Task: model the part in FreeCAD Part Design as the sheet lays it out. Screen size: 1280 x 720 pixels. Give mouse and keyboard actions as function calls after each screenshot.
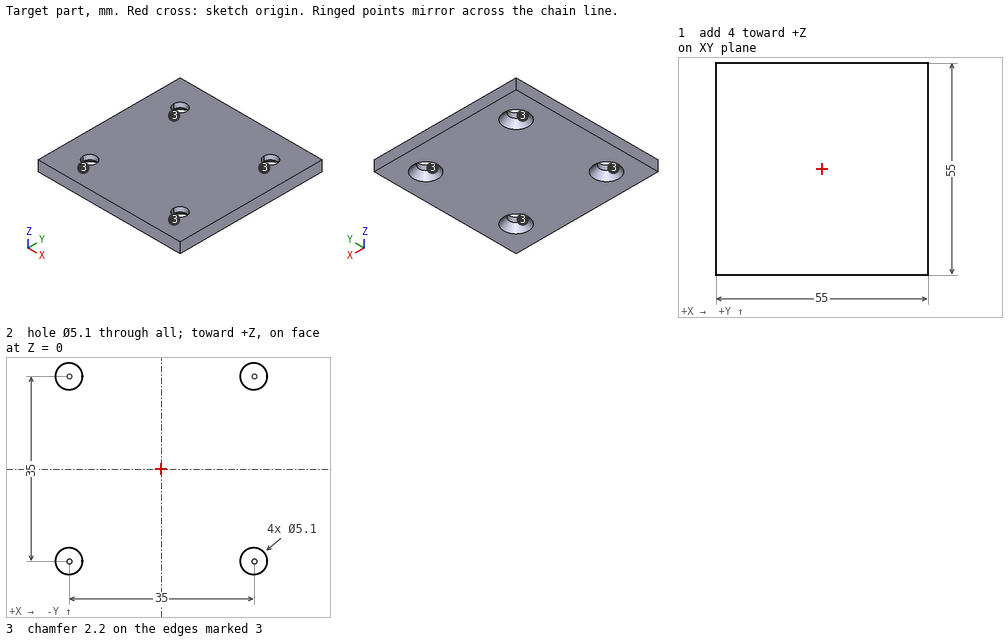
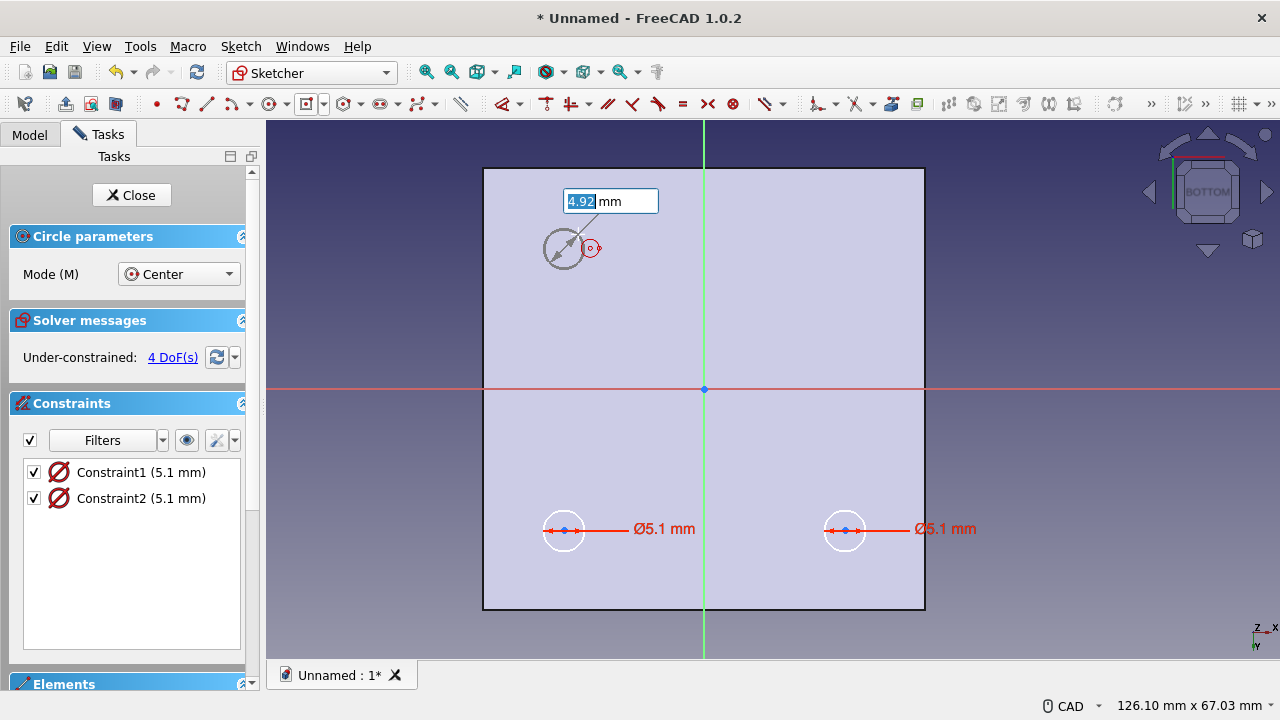
text(5.1)
key(Return)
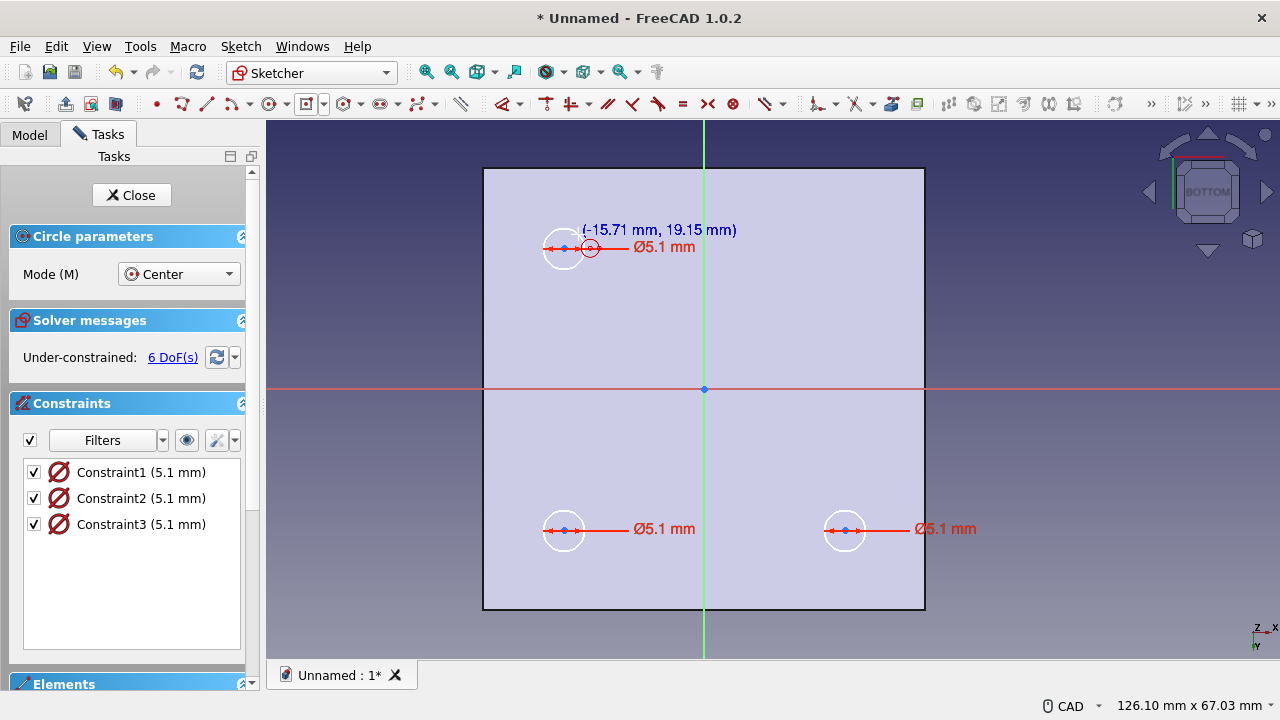
click(845, 248)
move(860, 234)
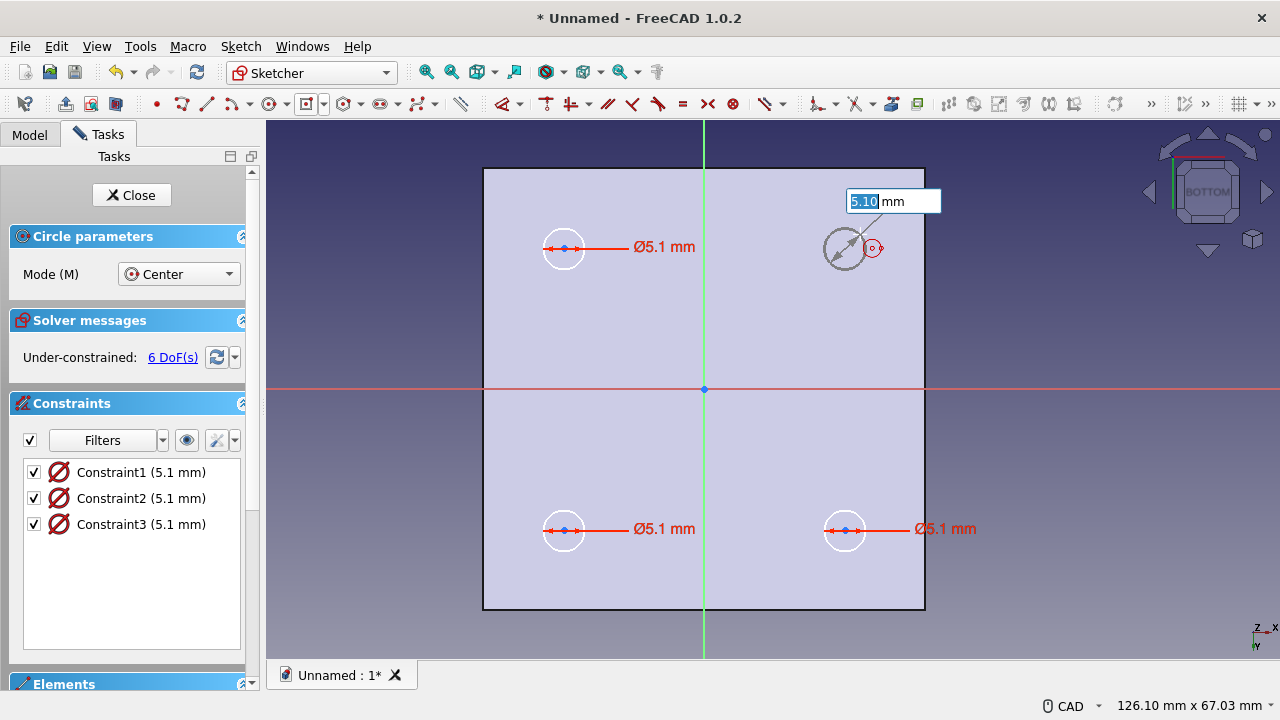
text(5.1)
key(Return)
key(Escape)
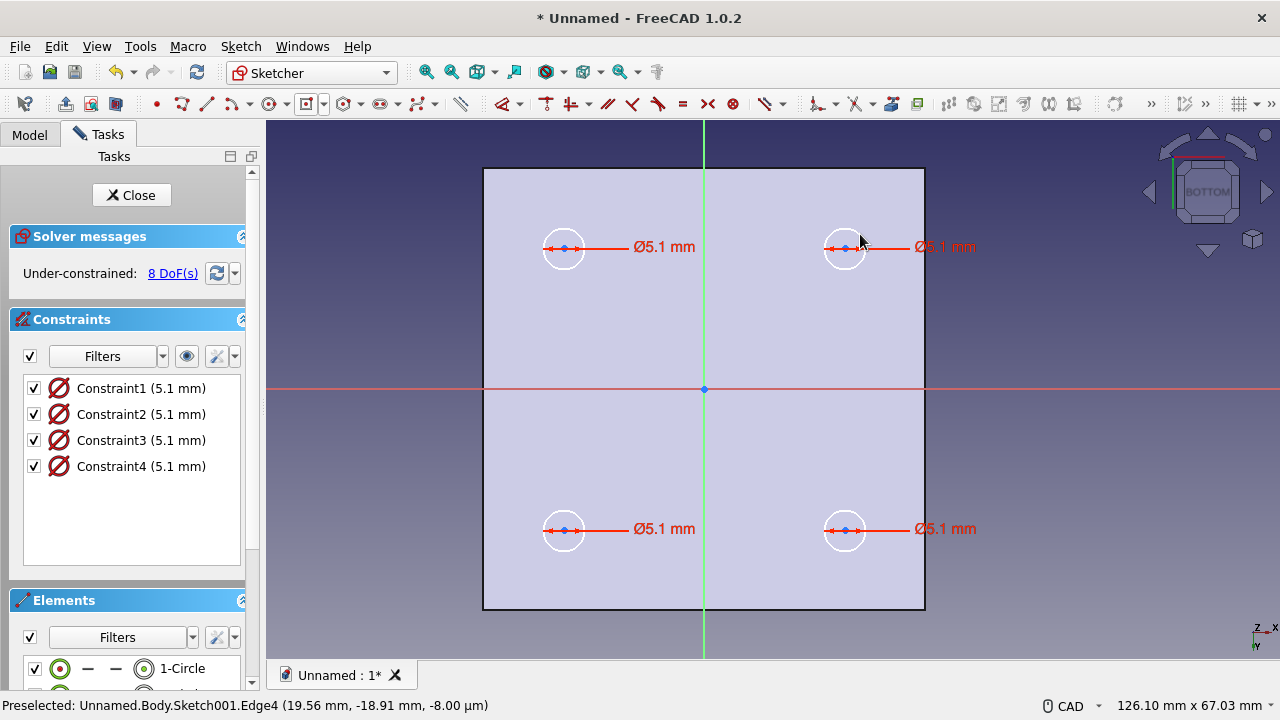
click(845, 531)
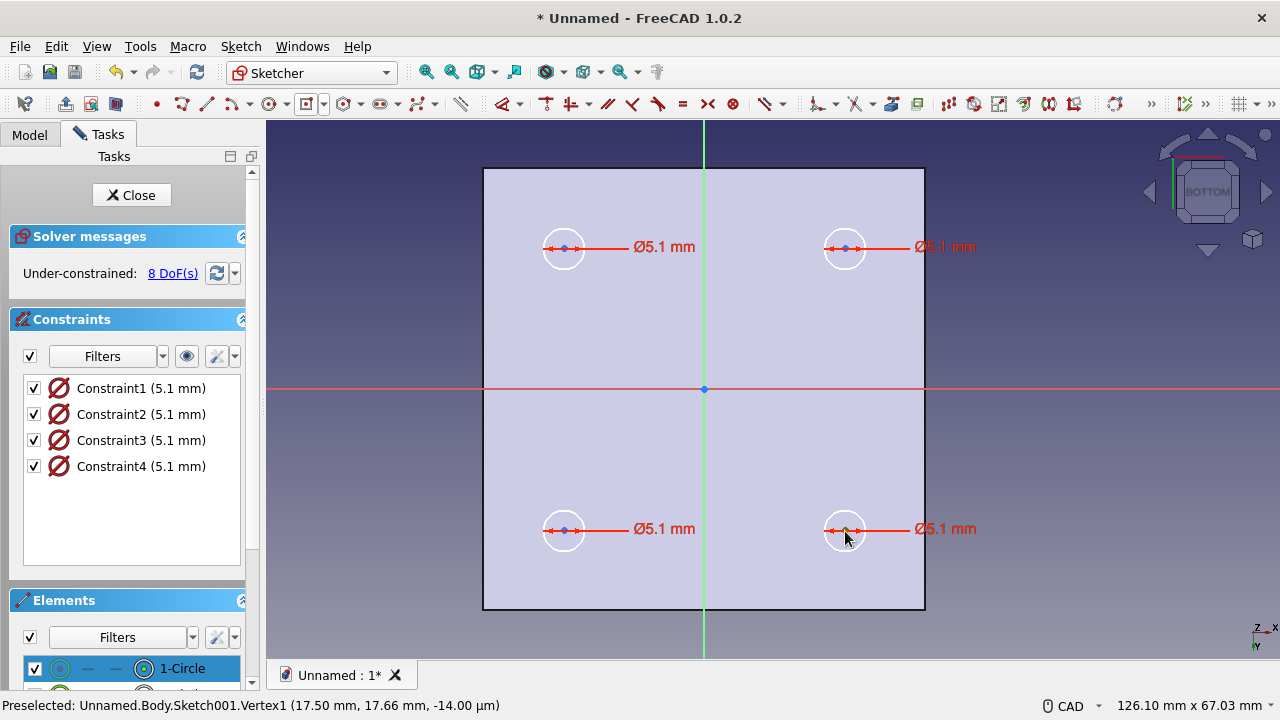
click(564, 531)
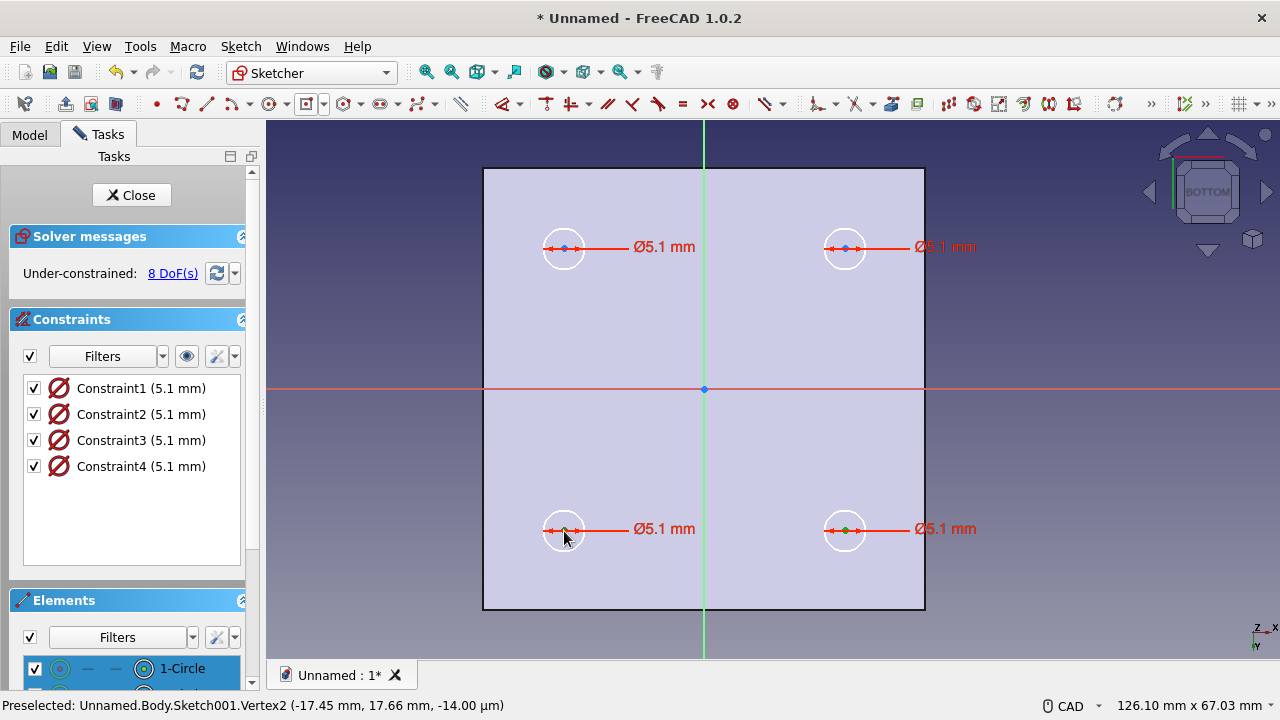
click(704, 596)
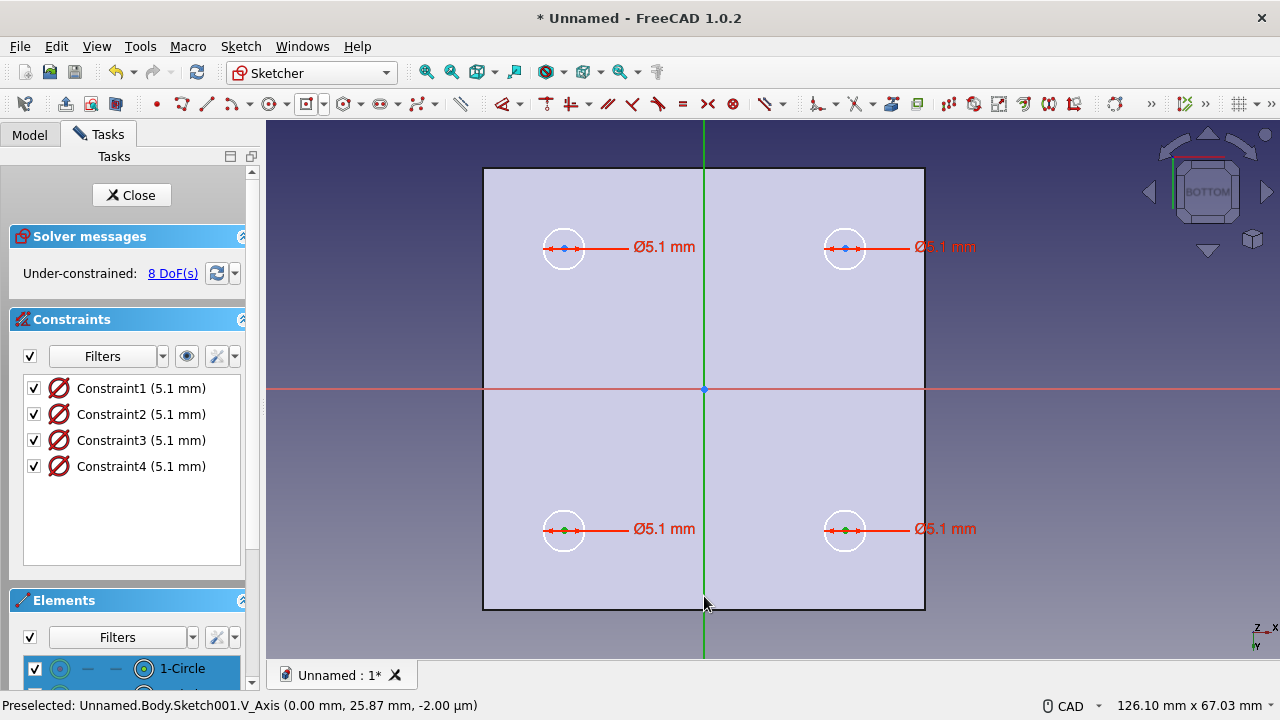
click(708, 104)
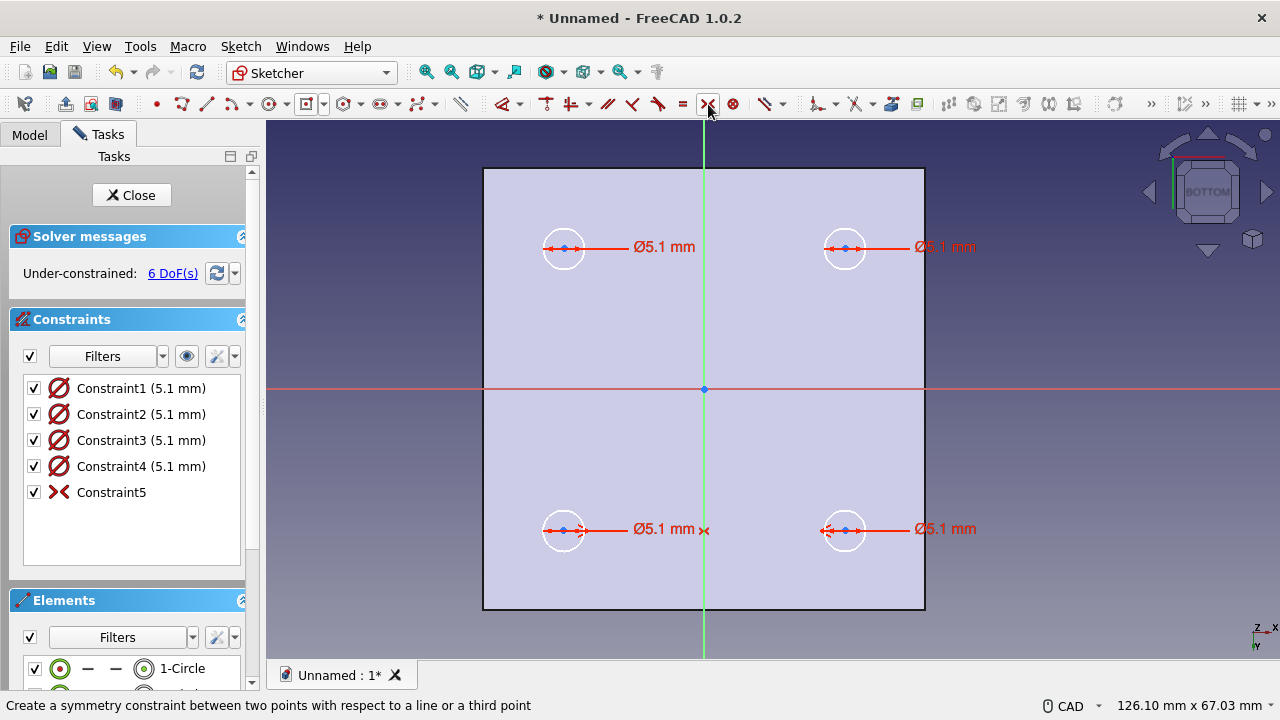
click(564, 531)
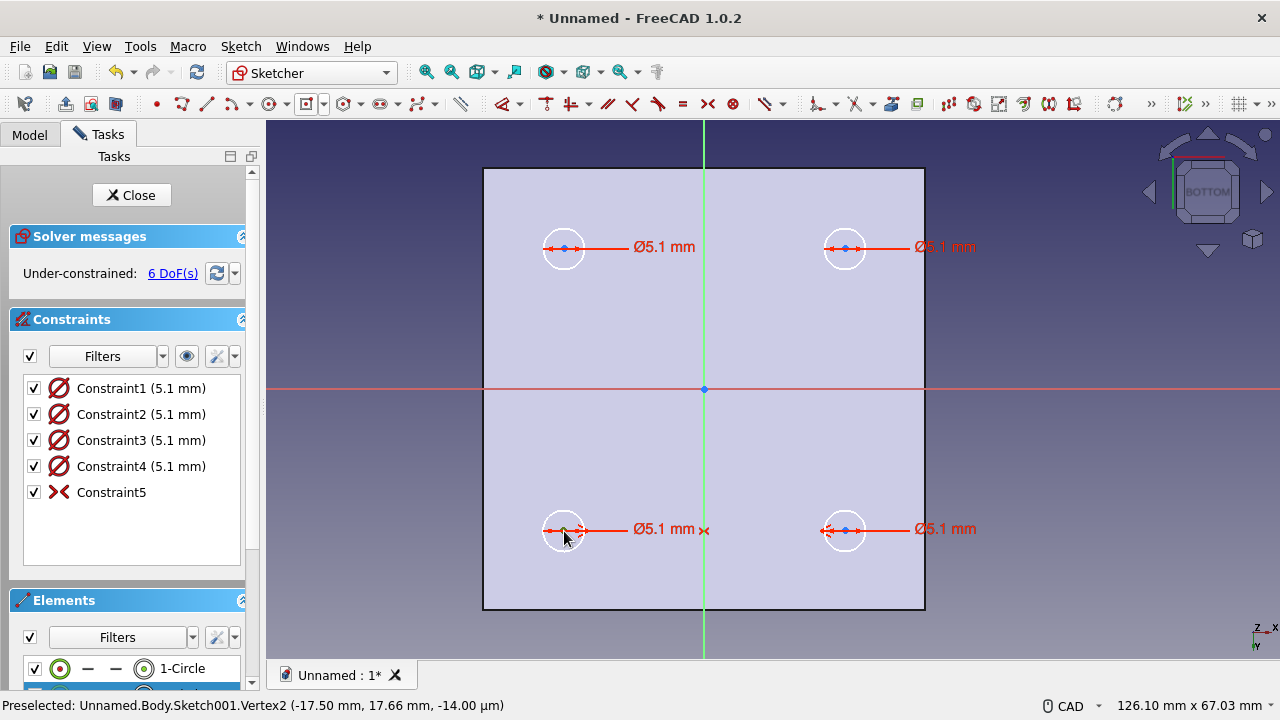
click(564, 249)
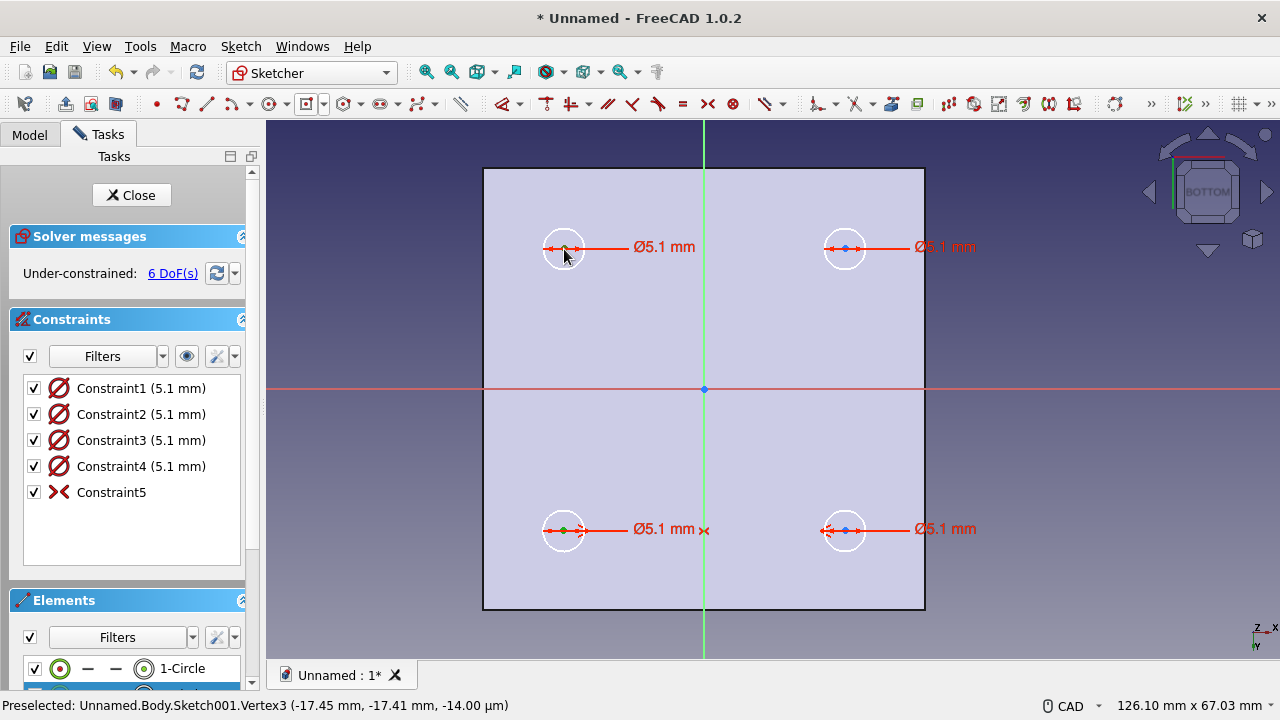
click(353, 389)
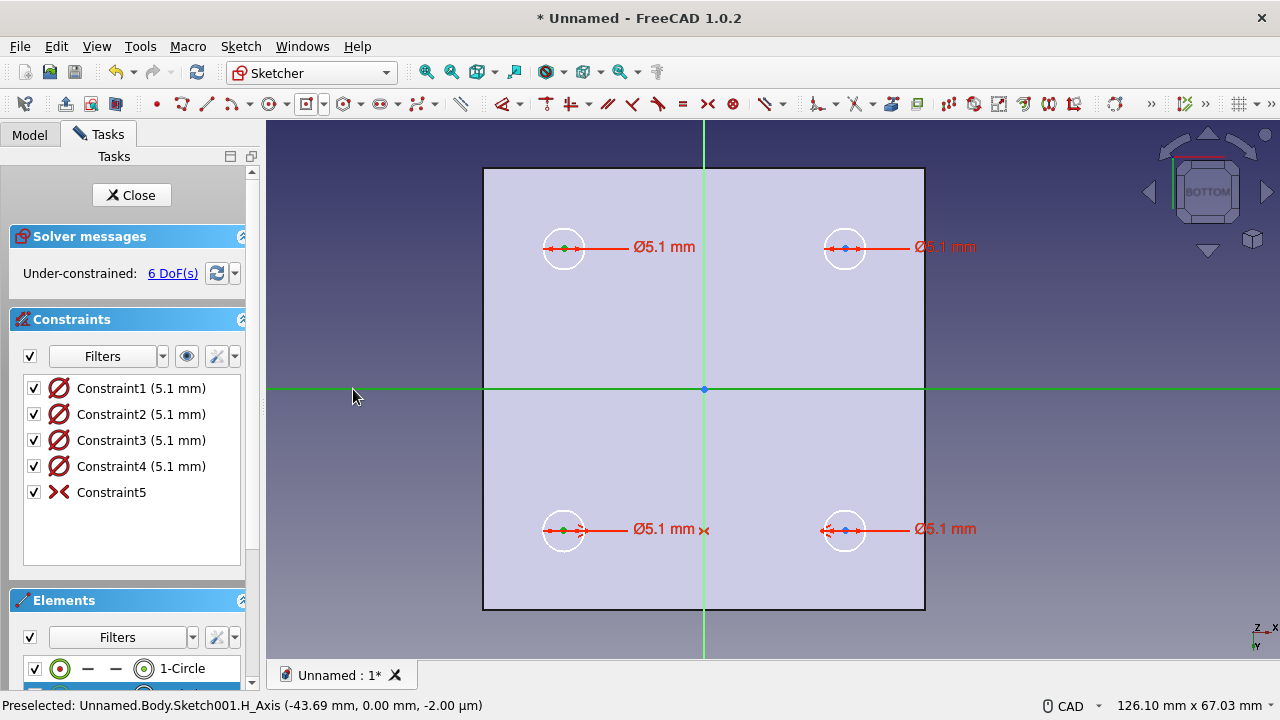
click(708, 104)